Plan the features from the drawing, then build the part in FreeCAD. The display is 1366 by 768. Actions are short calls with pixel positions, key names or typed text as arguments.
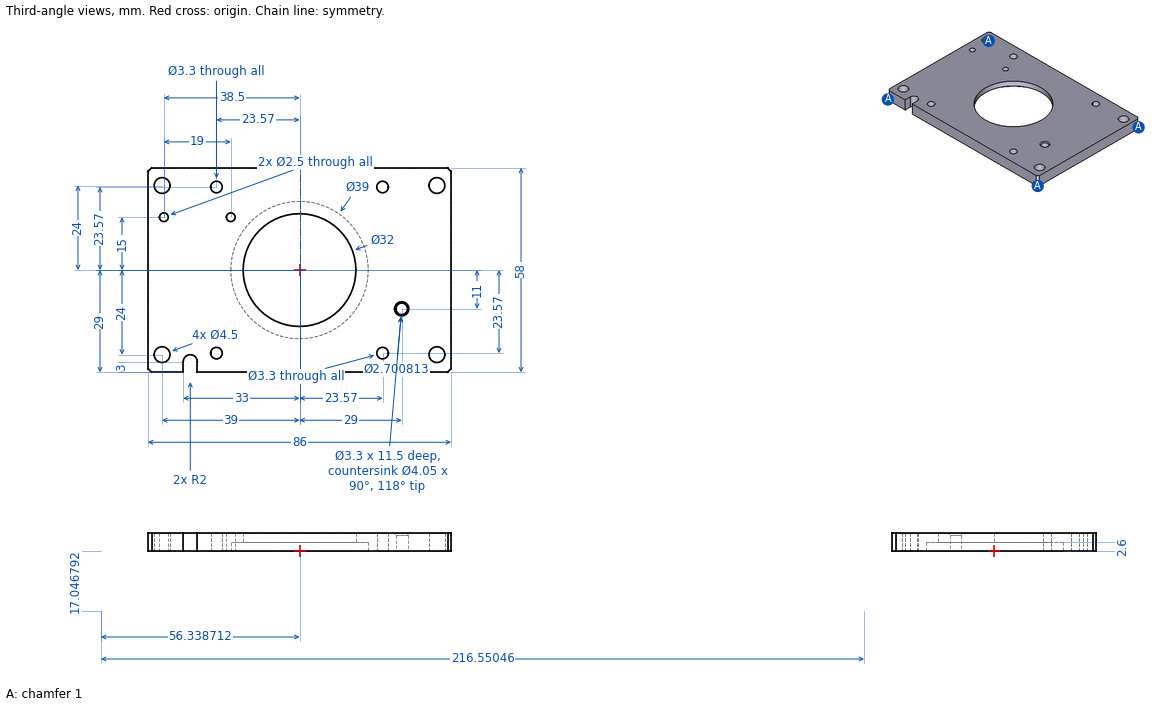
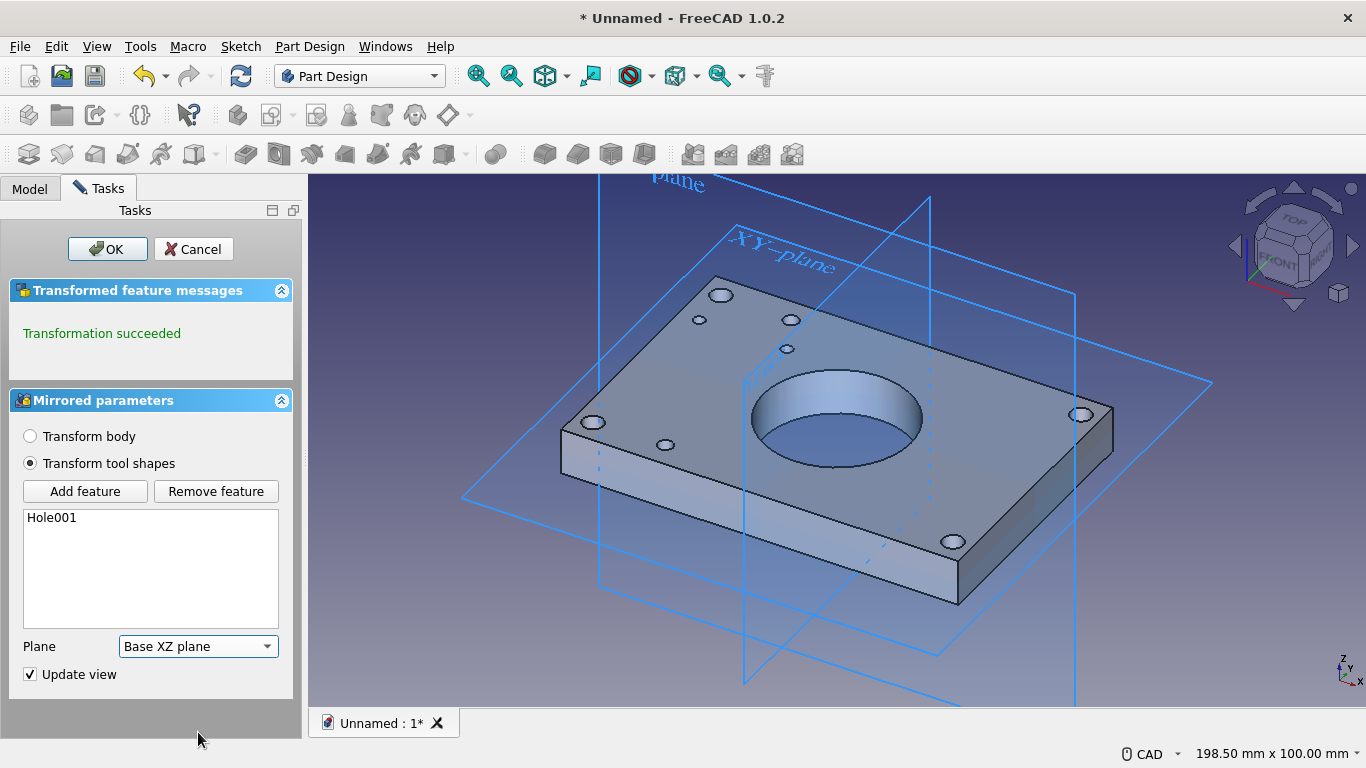
click(108, 249)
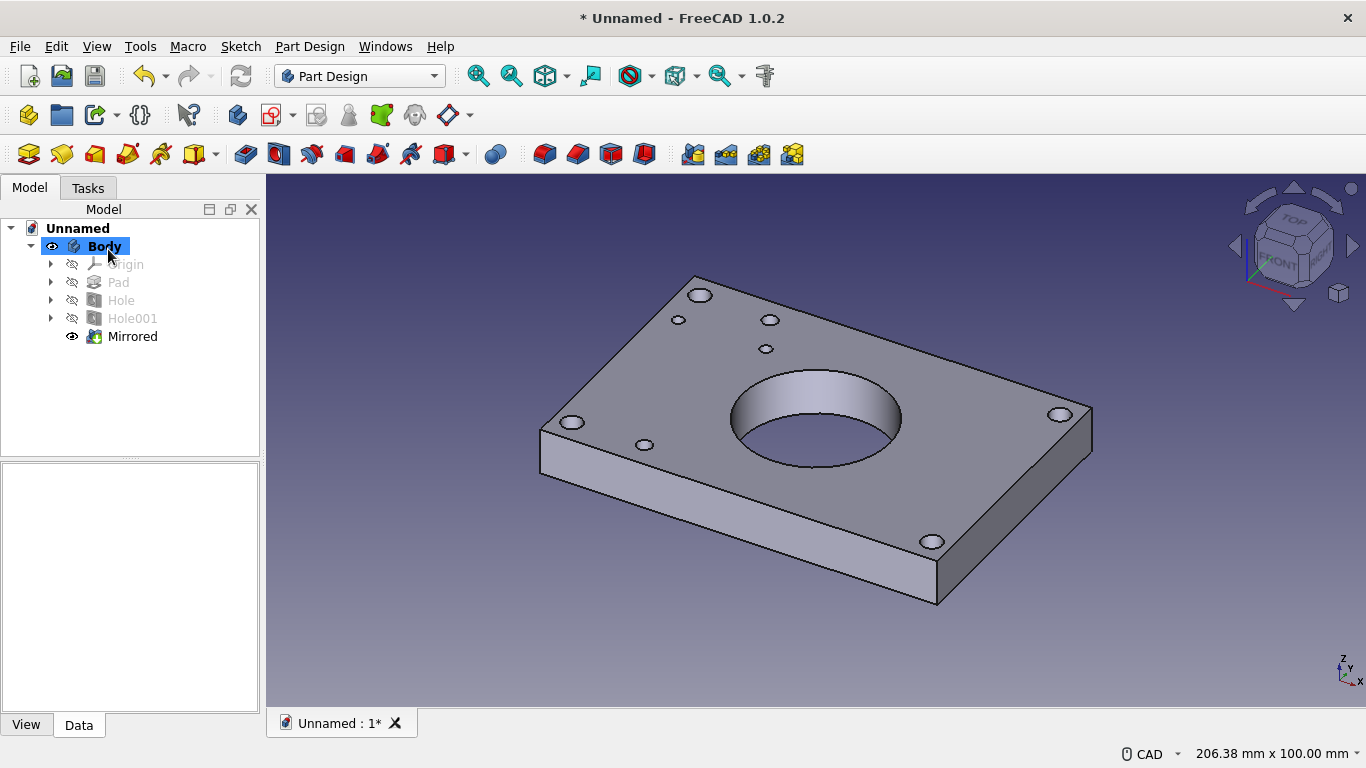
click(117, 318)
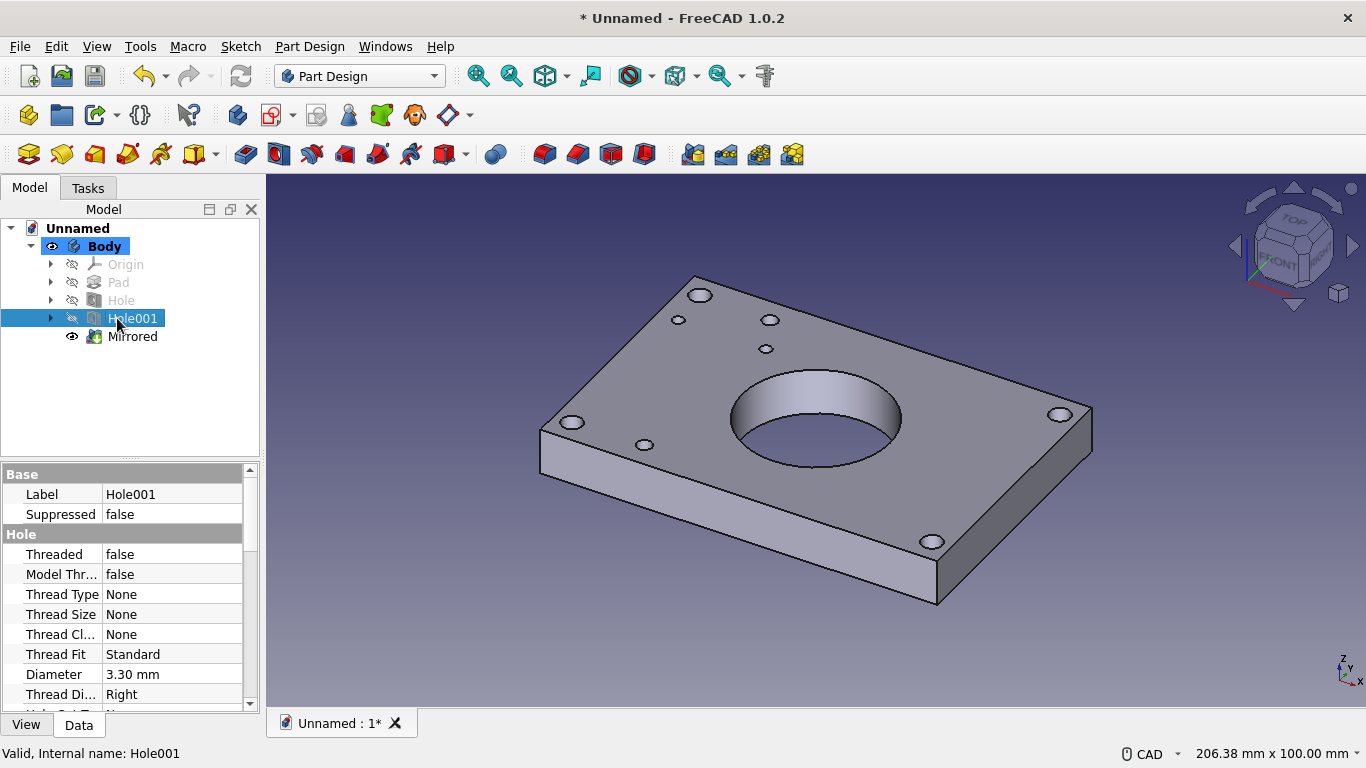
click(693, 154)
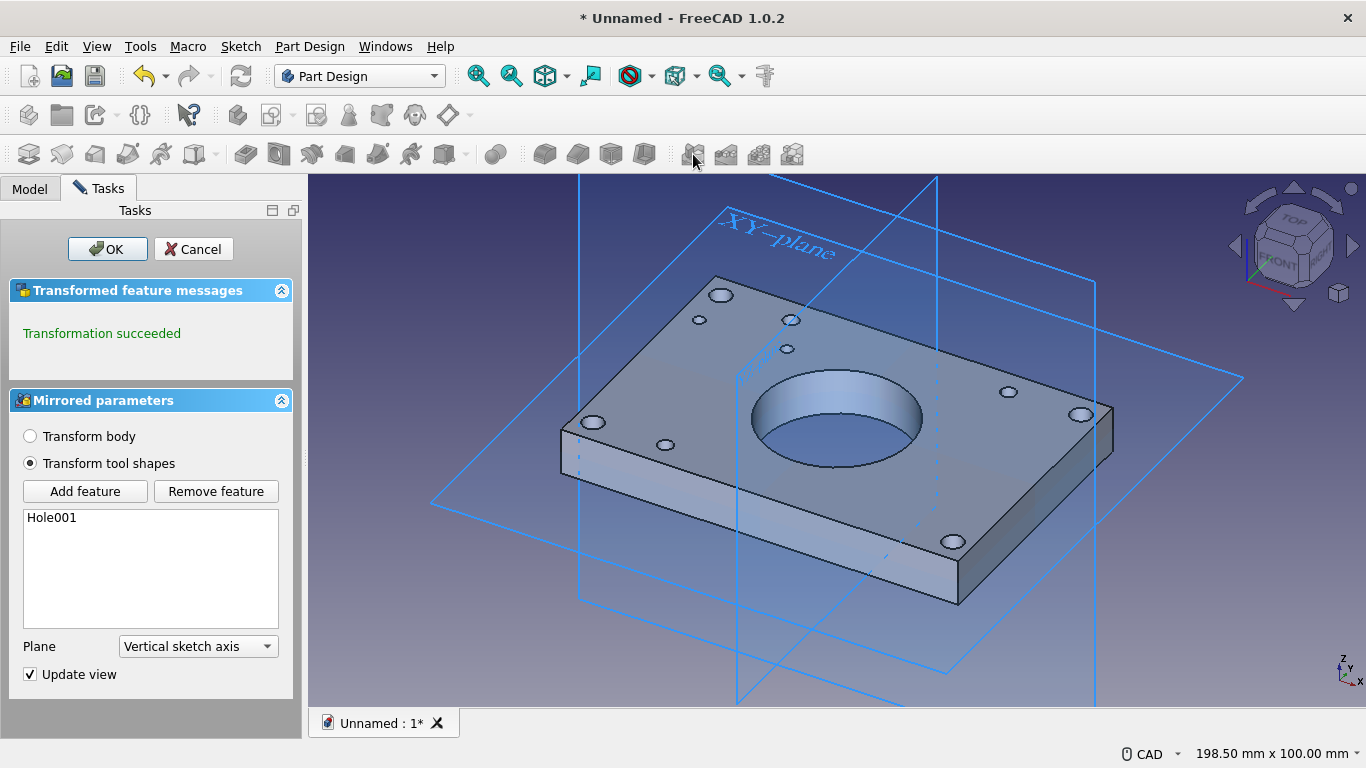
click(199, 646)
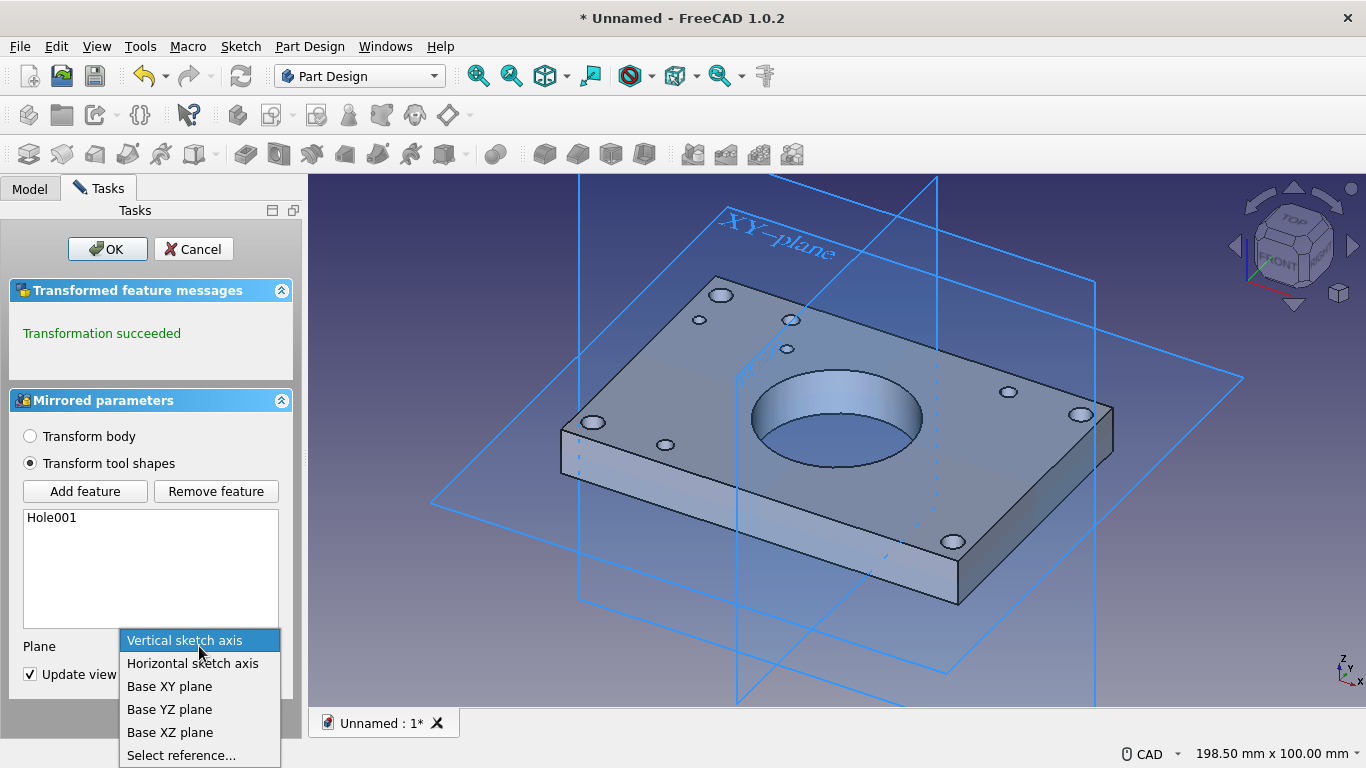
click(198, 710)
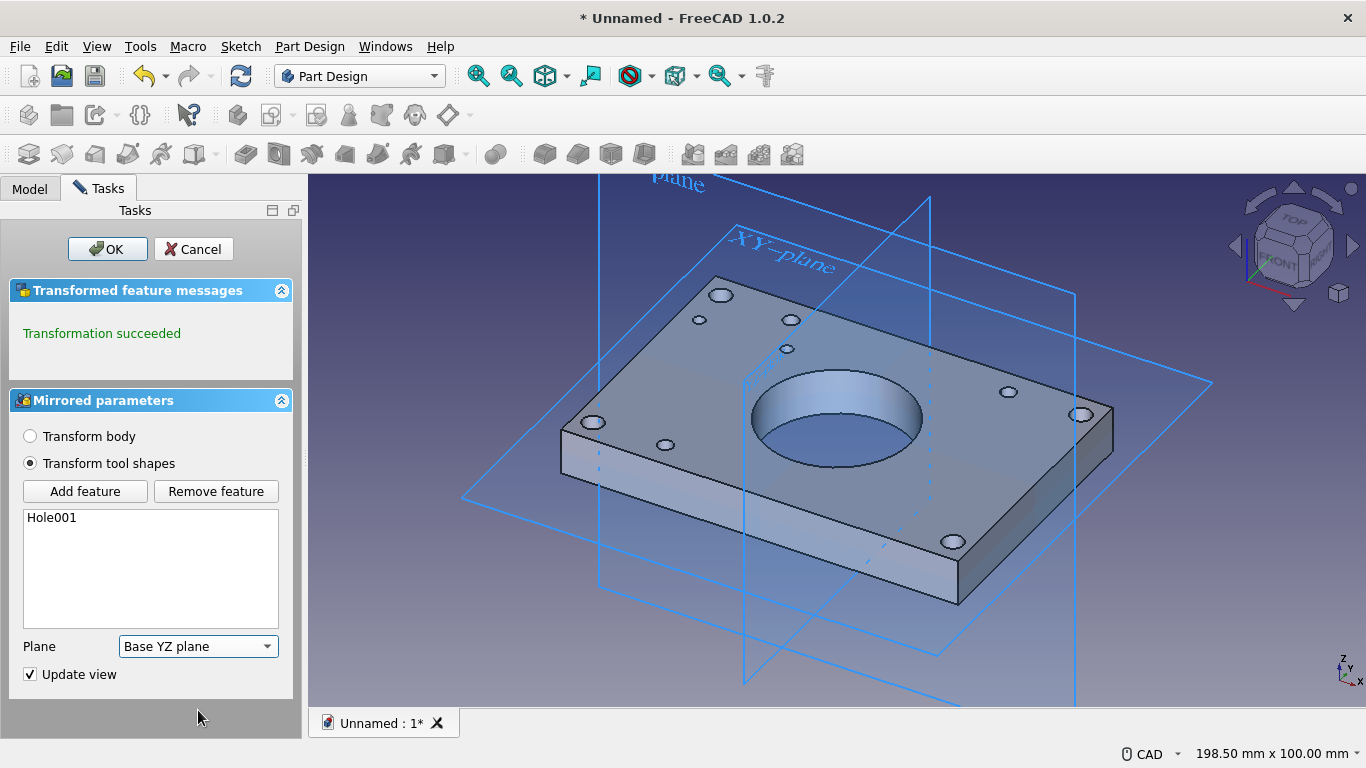
click(108, 249)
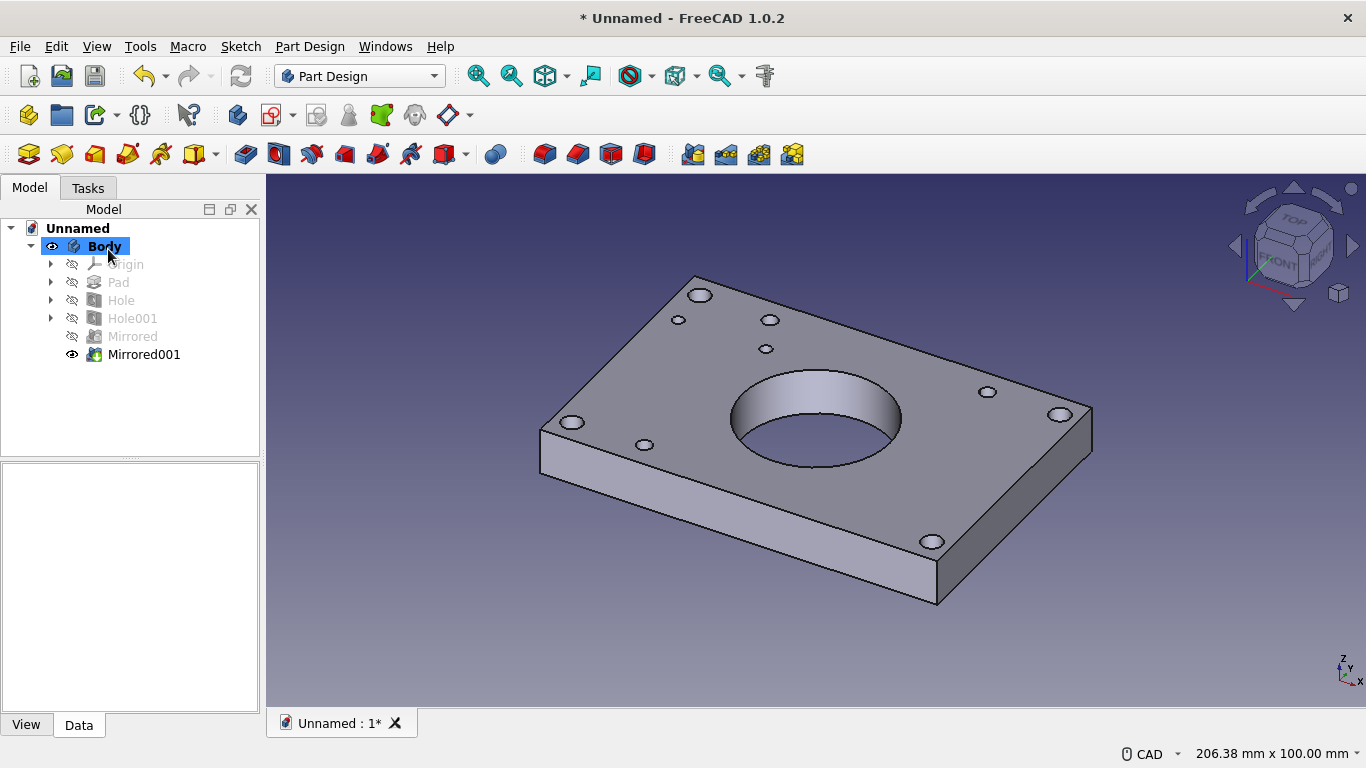
click(885, 499)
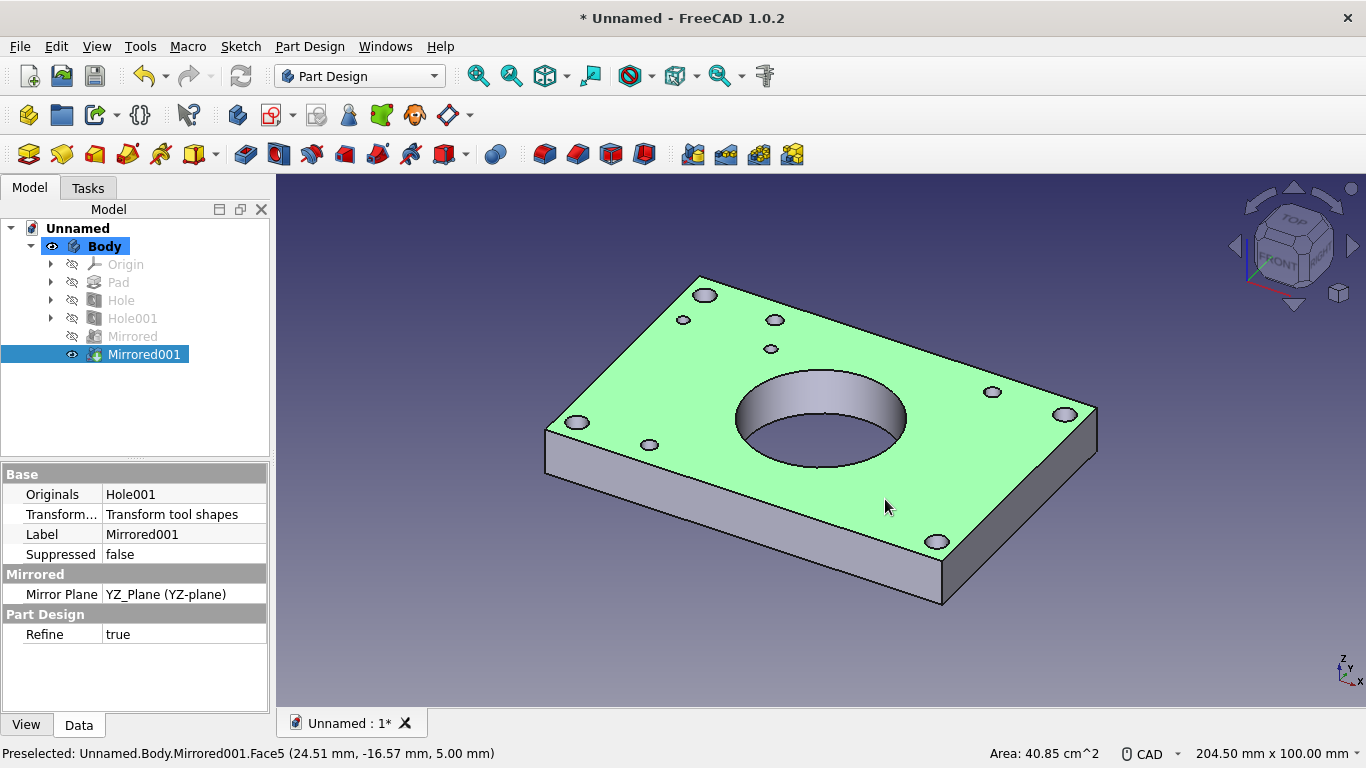
click(270, 116)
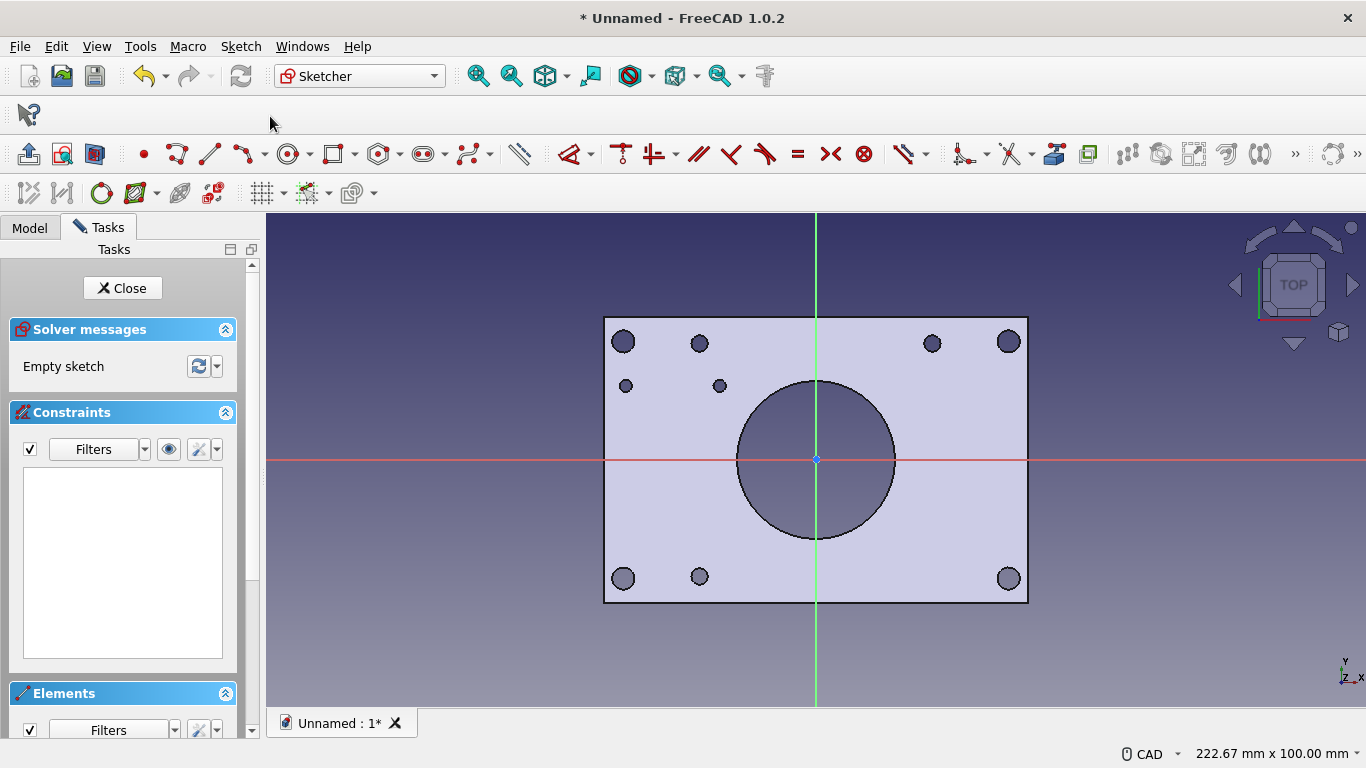
scroll(942, 583, up, 15)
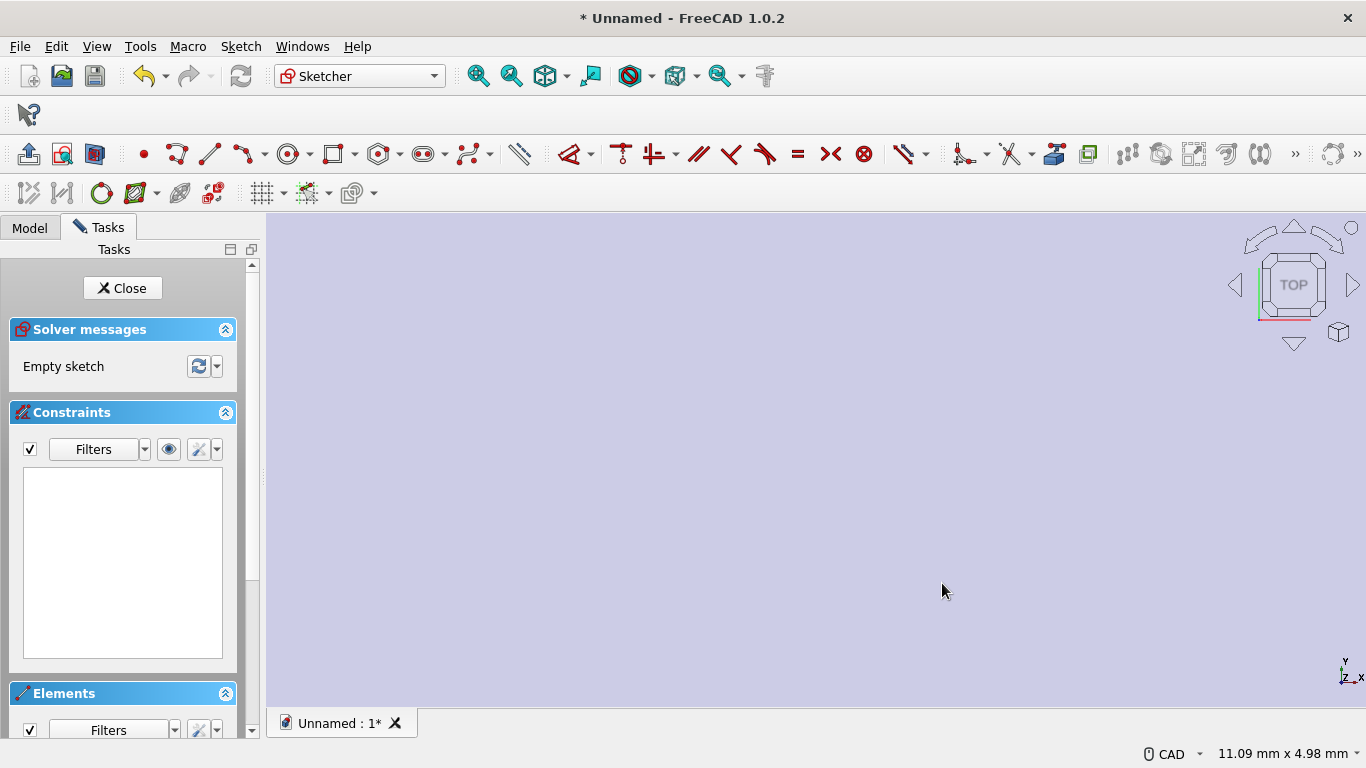
key(g)
key(c)